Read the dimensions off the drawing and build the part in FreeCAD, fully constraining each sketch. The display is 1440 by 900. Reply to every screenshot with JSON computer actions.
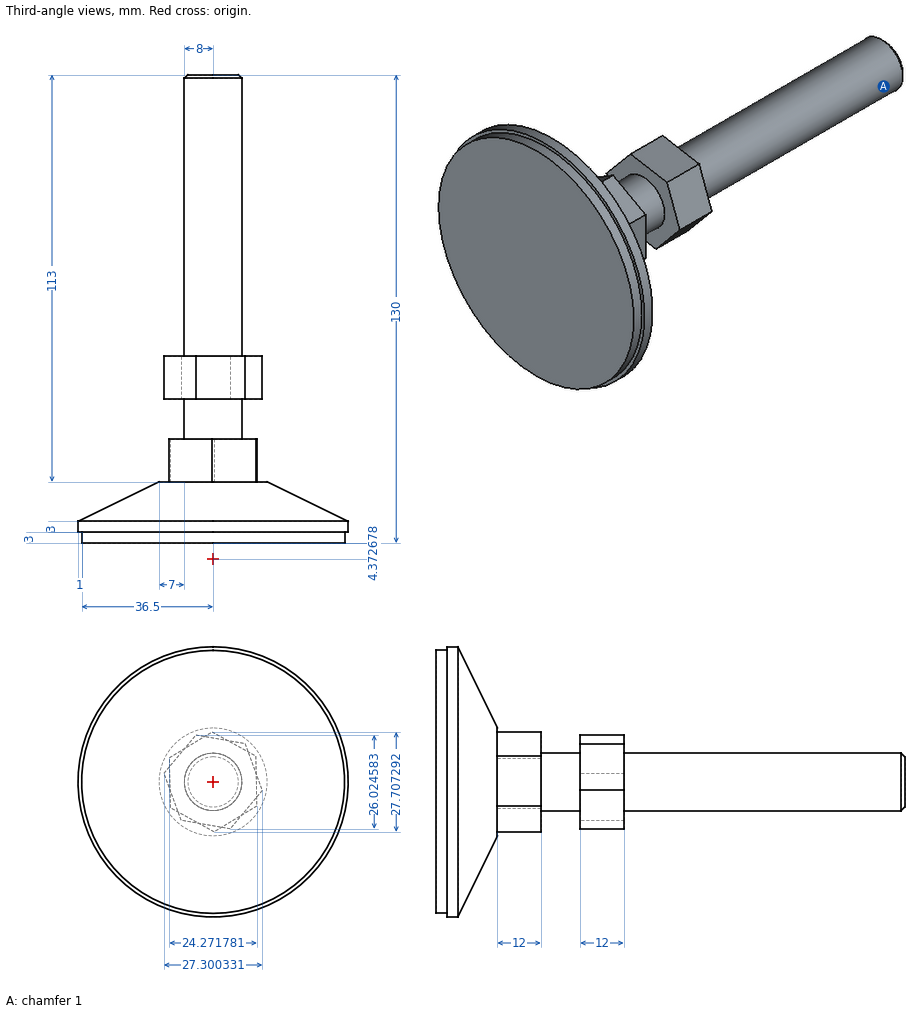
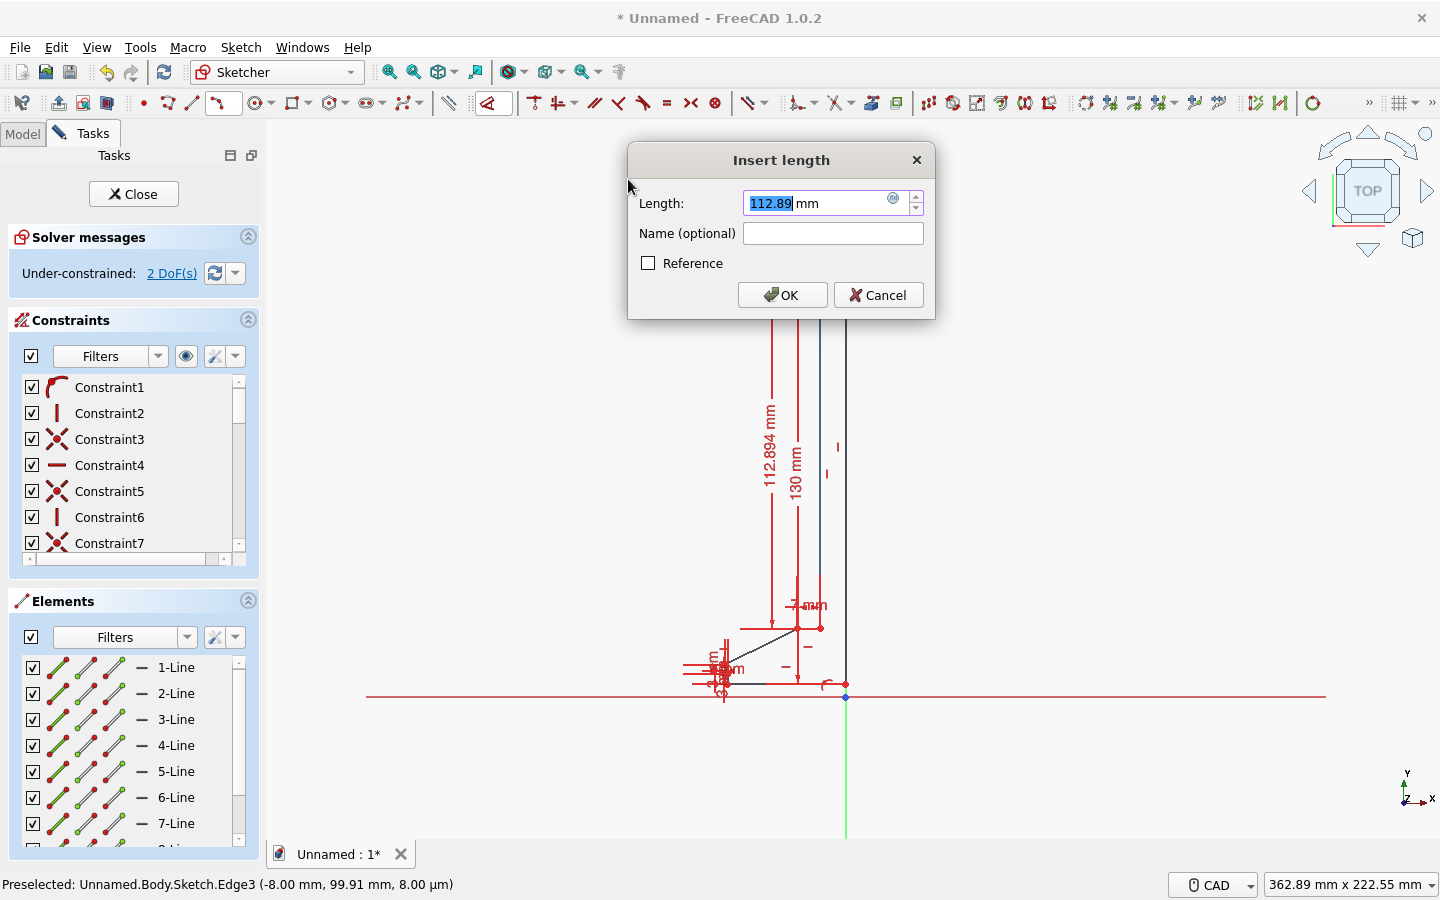
{"action": "type", "text": "113"}
{"action": "key", "text": "Return"}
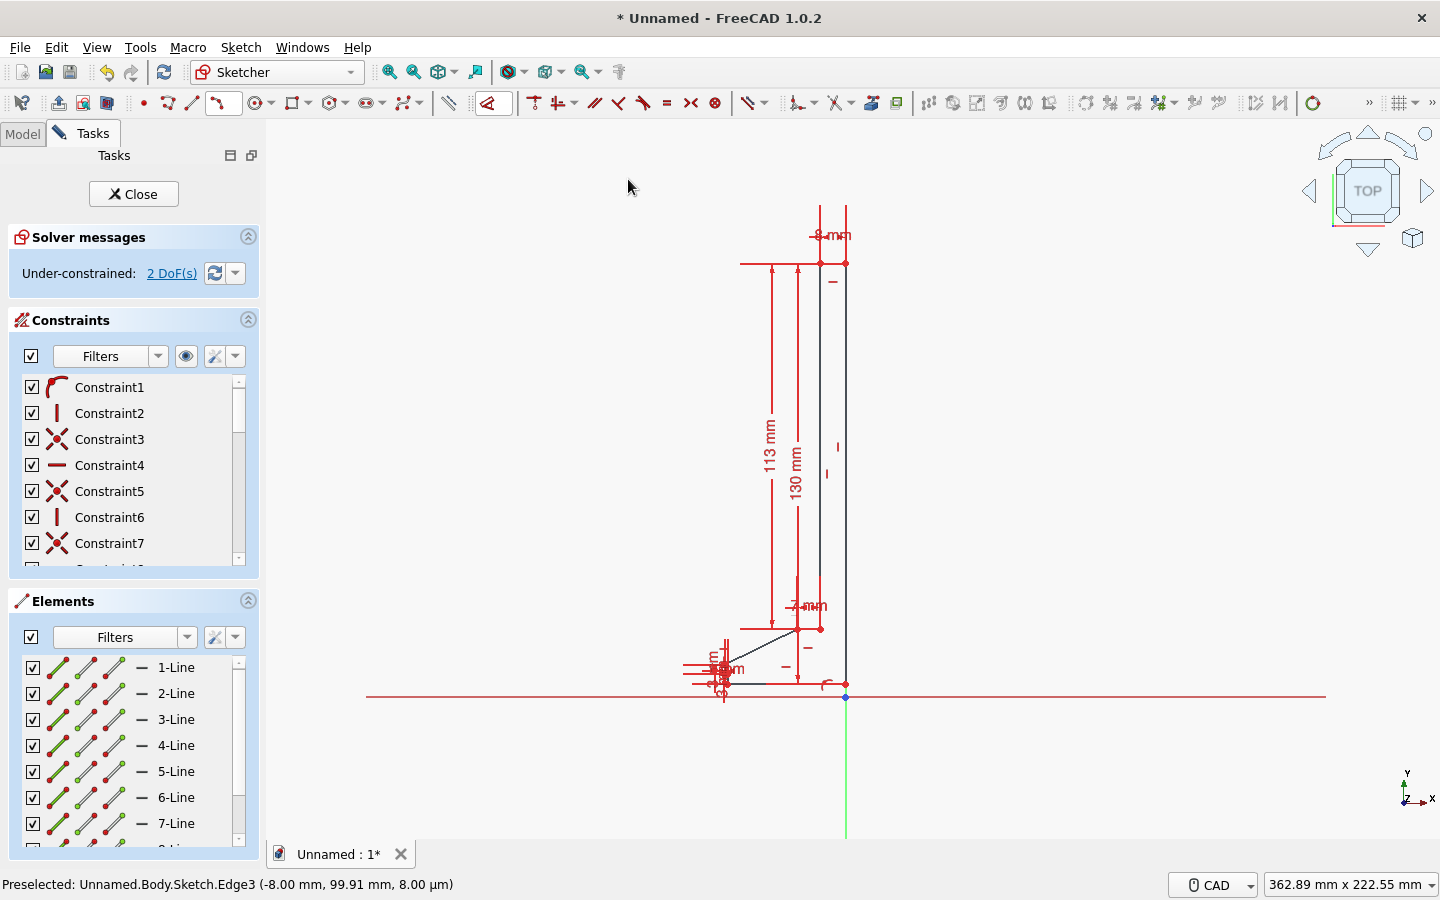
{"action": "left_click", "coordinate": [763, 684]}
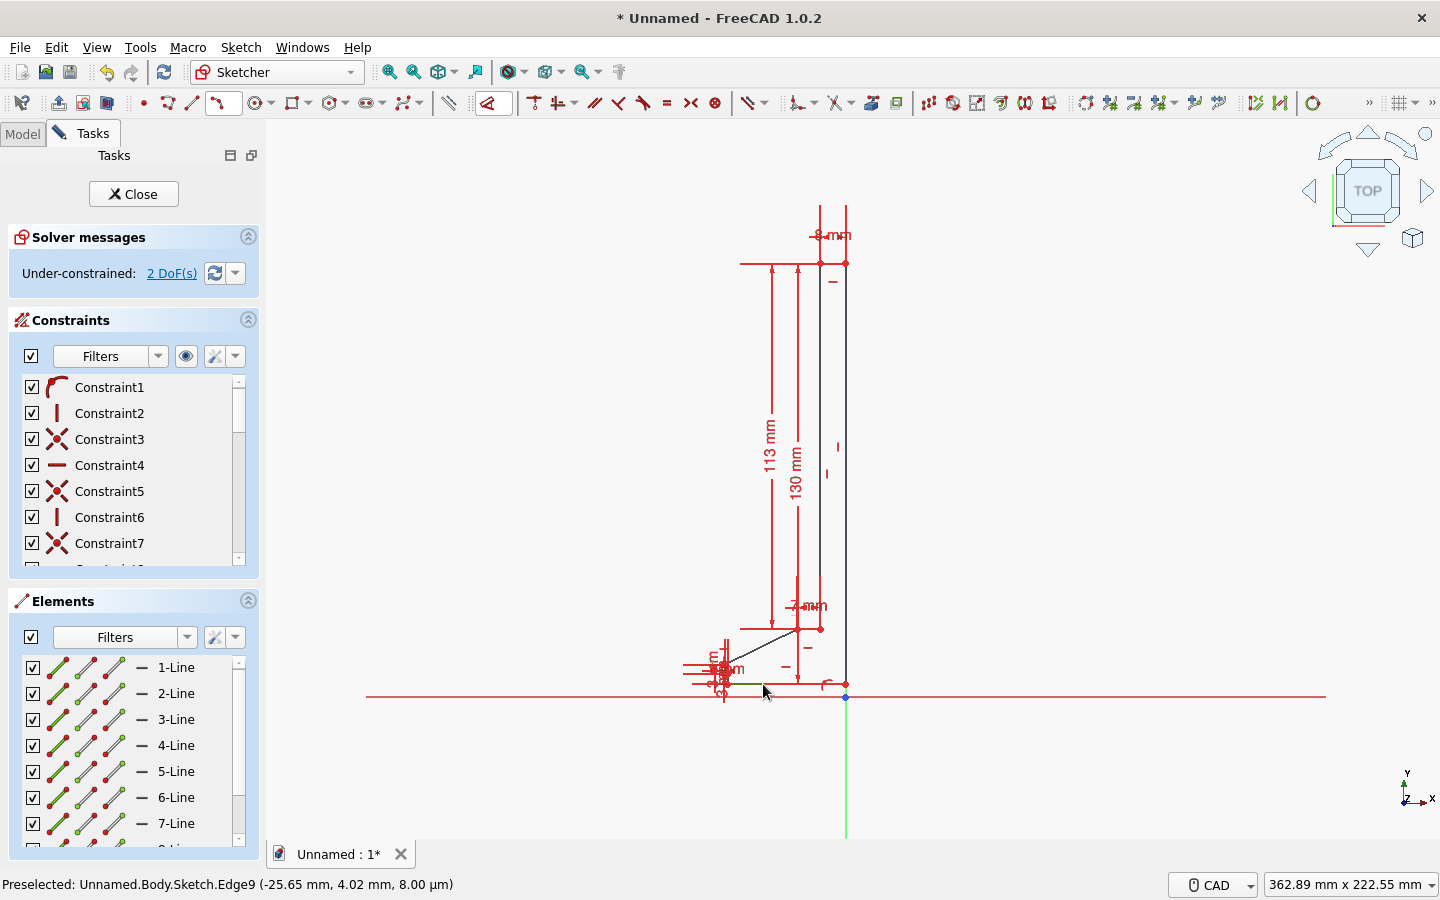
{"action": "left_click", "coordinate": [506, 104]}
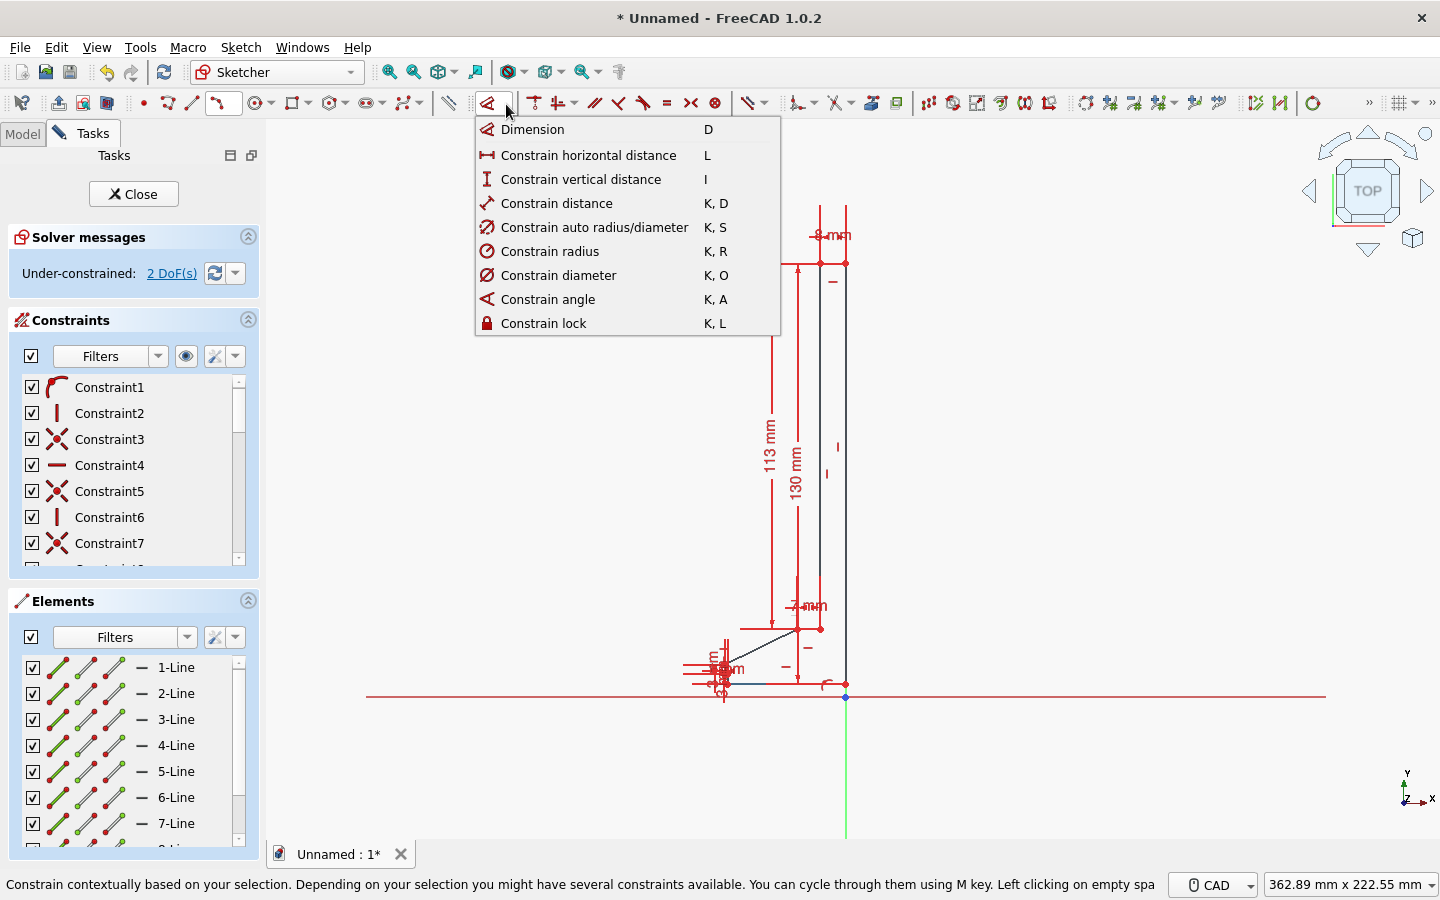
{"action": "left_click", "coordinate": [628, 155]}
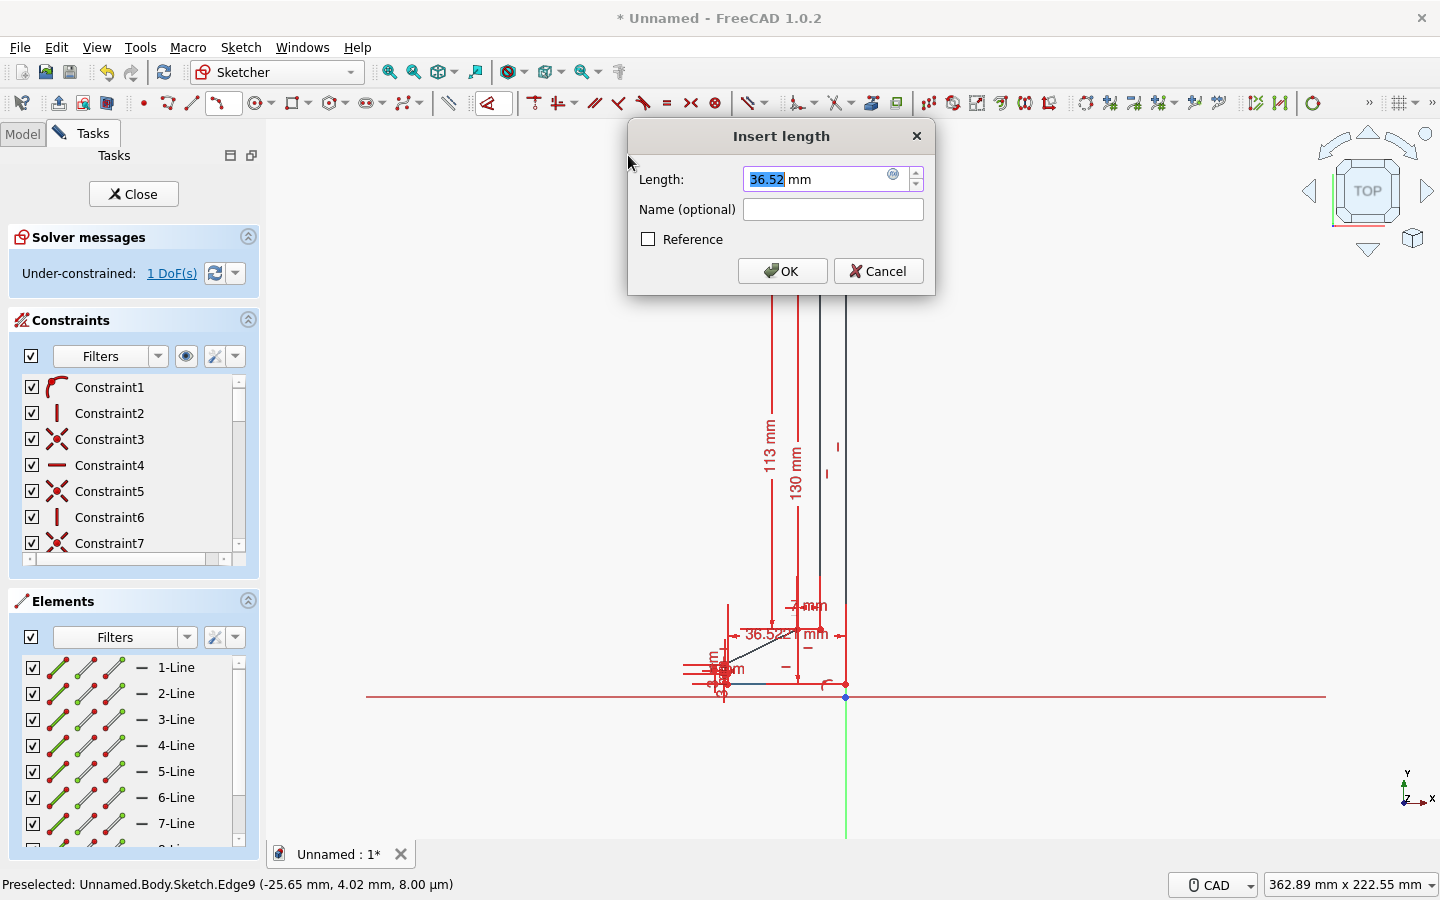
{"action": "type", "text": "36.5"}
{"action": "key", "text": "Return"}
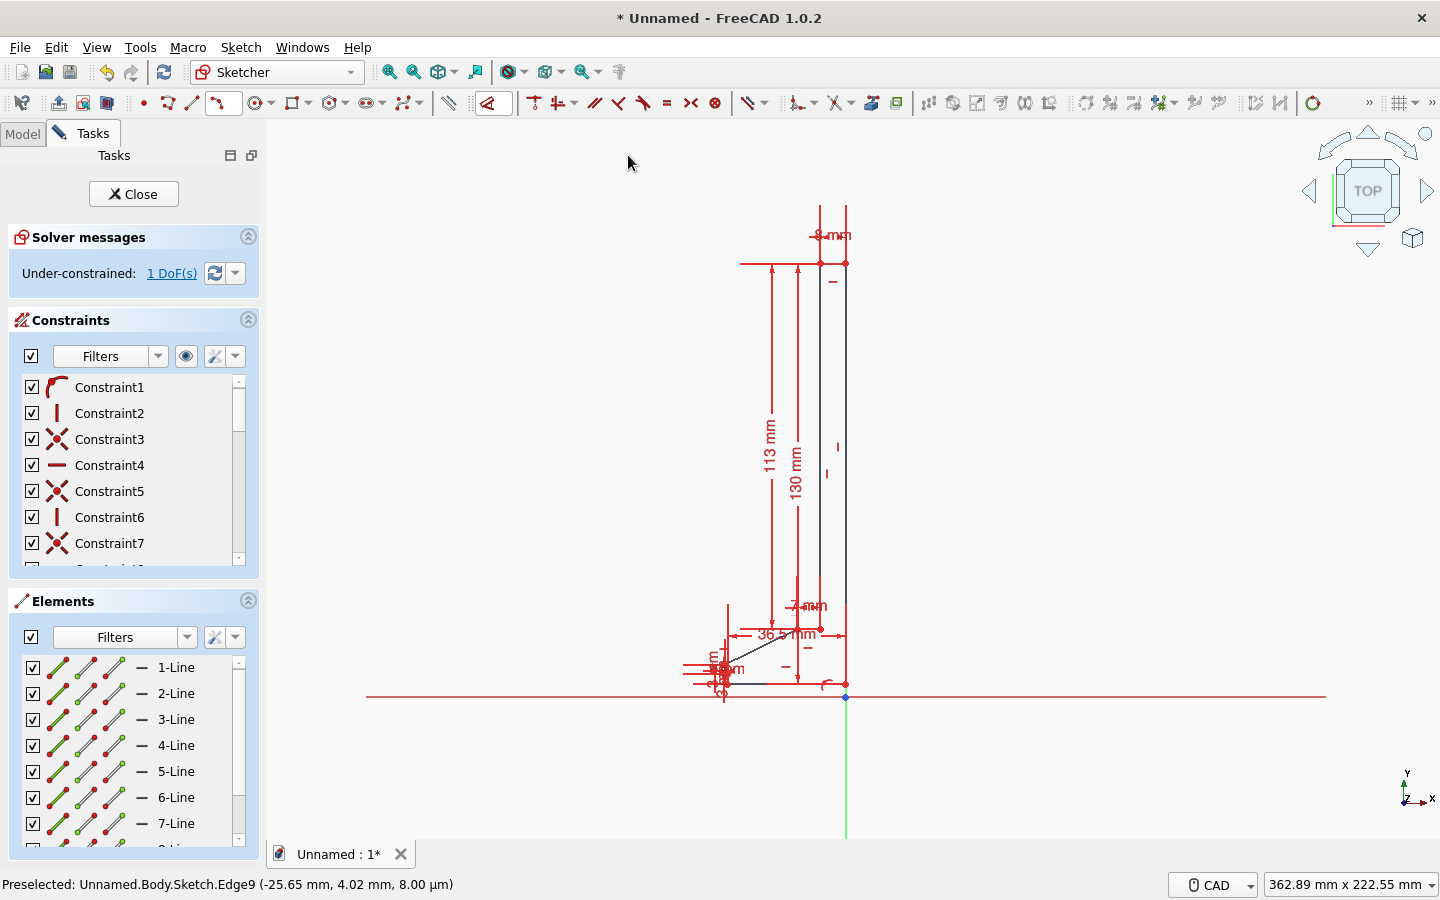
{"action": "scroll", "coordinate": [846, 684], "scroll_direction": "up", "scroll_amount": 6}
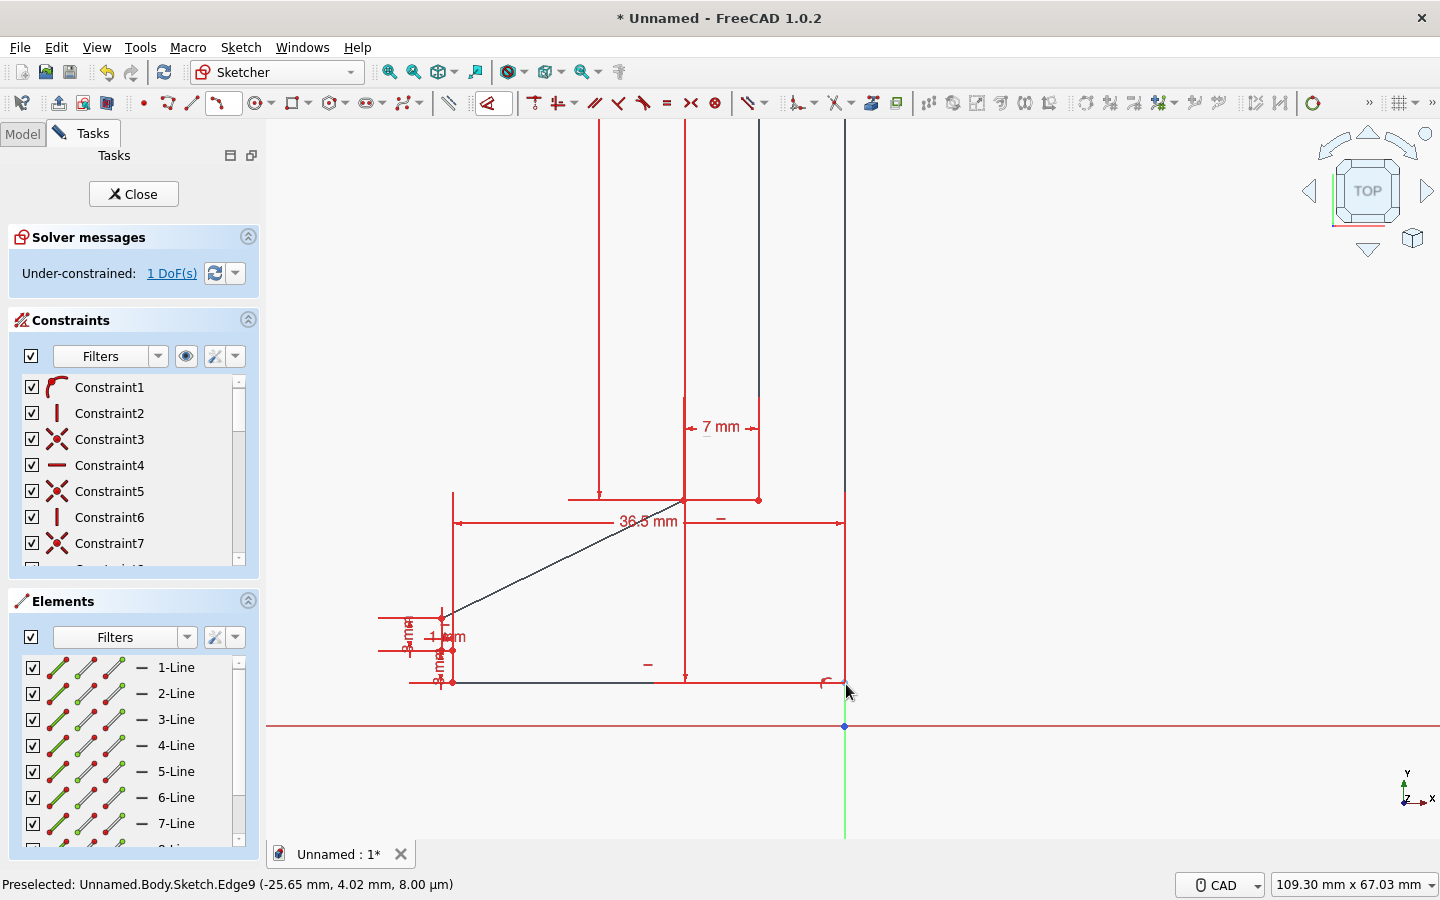
{"action": "left_click", "coordinate": [845, 683]}